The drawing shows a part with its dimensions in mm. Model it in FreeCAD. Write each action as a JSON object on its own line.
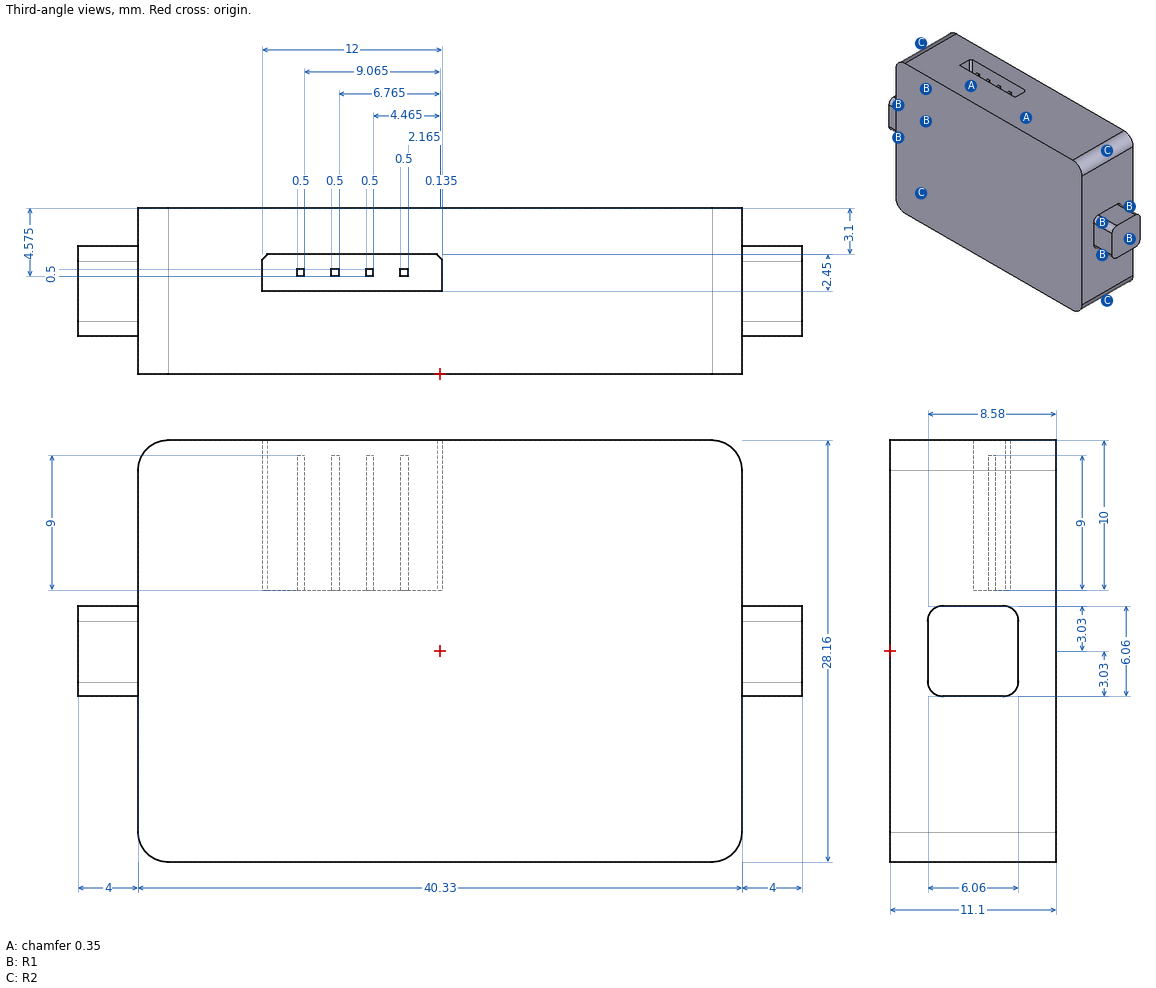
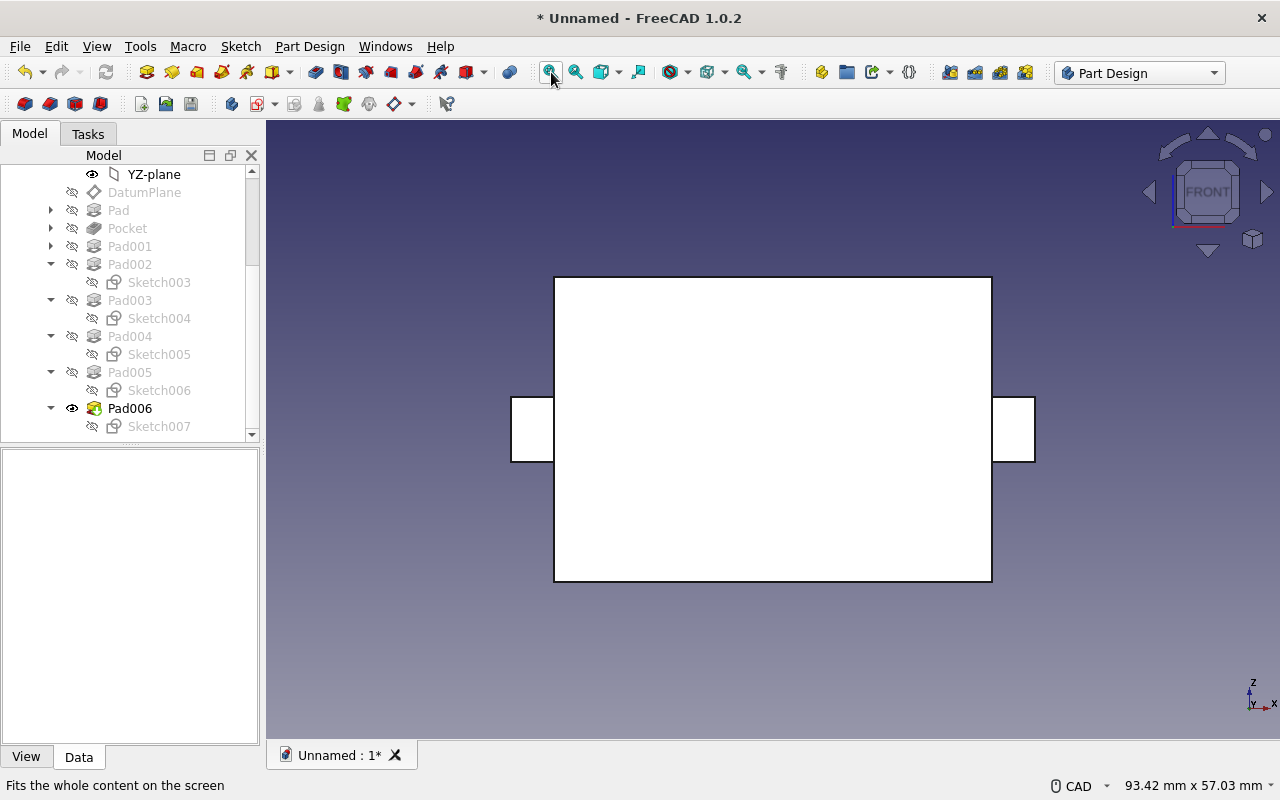
{"action": "key", "text": "3"}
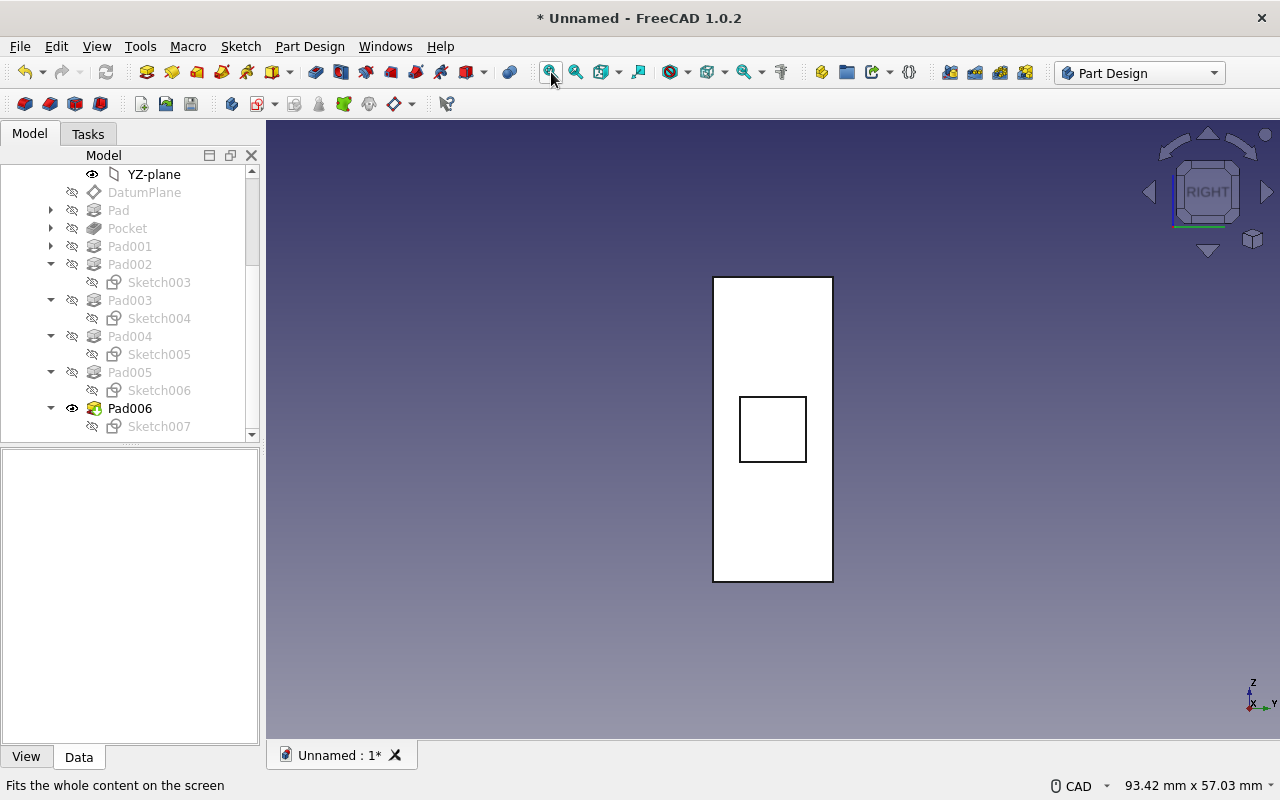
{"action": "key", "text": "5"}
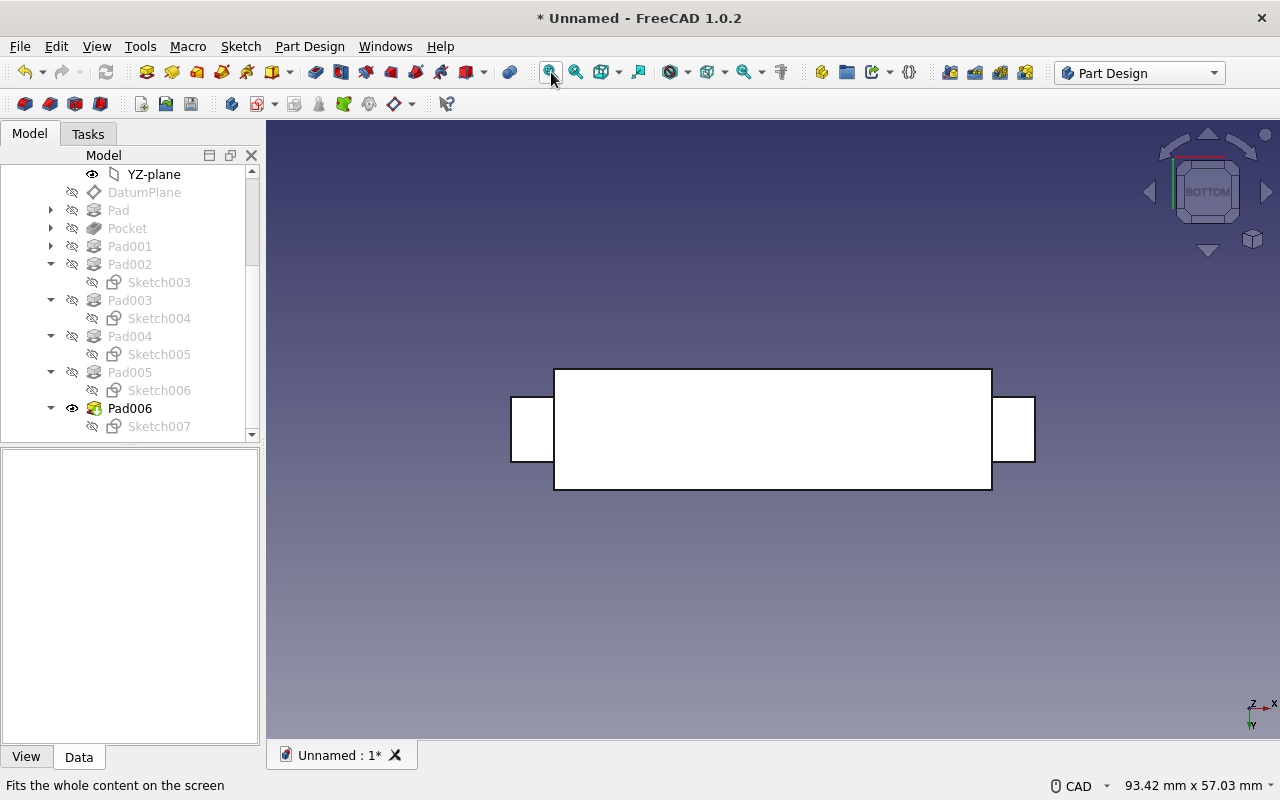
{"action": "key", "text": "4"}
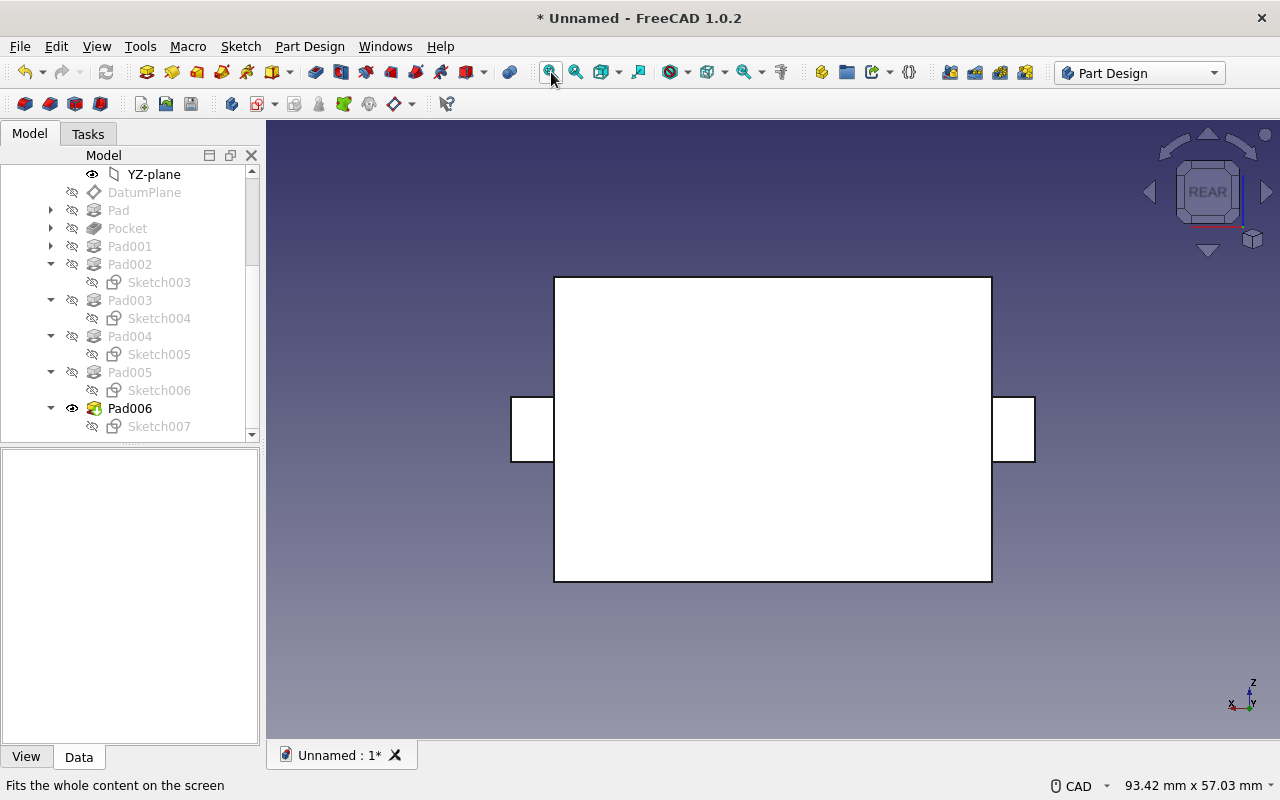
{"action": "key", "text": "6"}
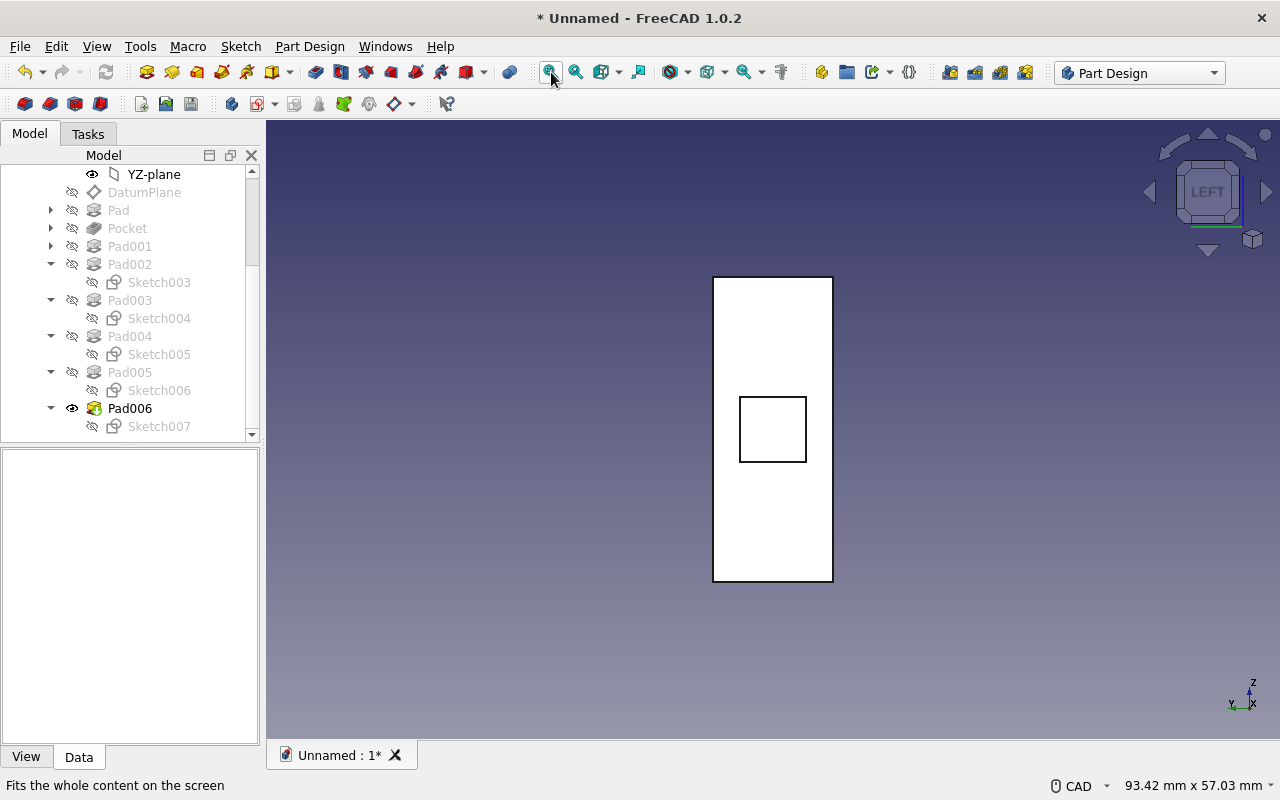
{"action": "key", "text": "v 3"}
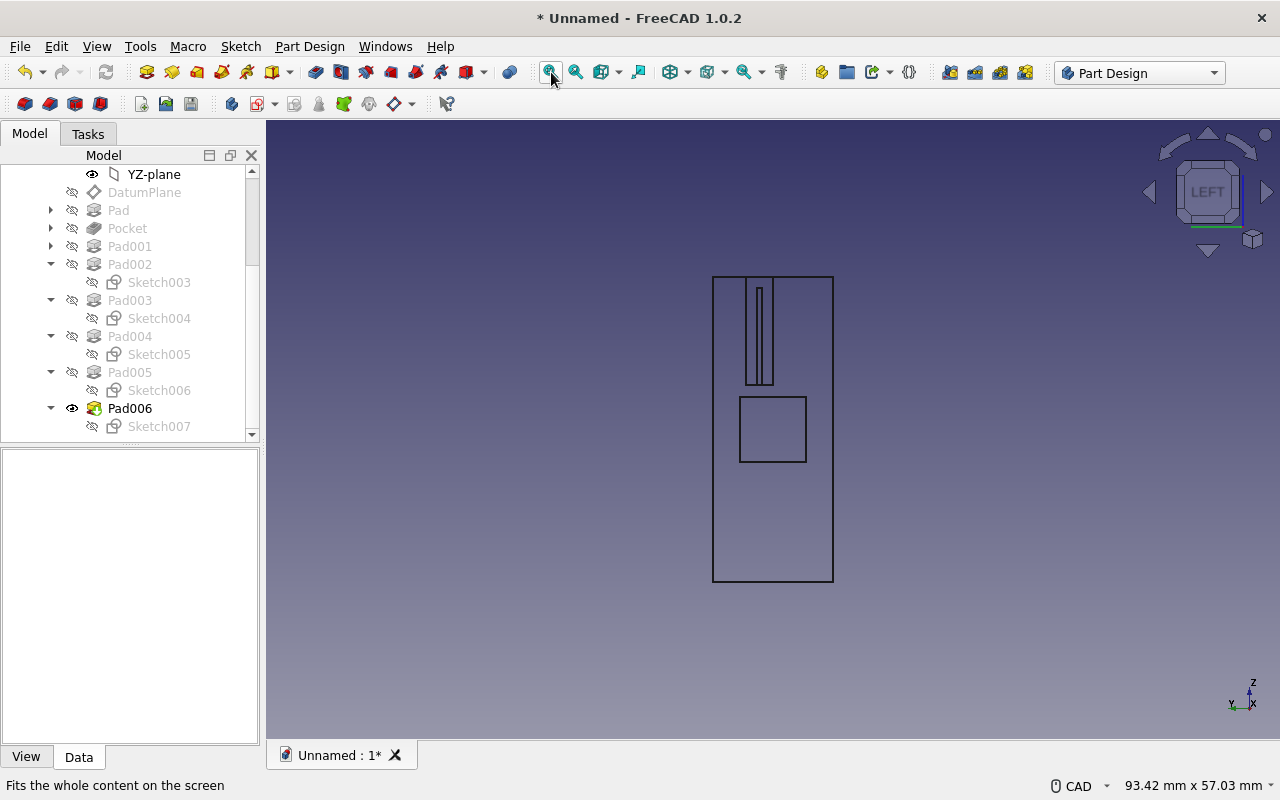
{"action": "key", "text": "0"}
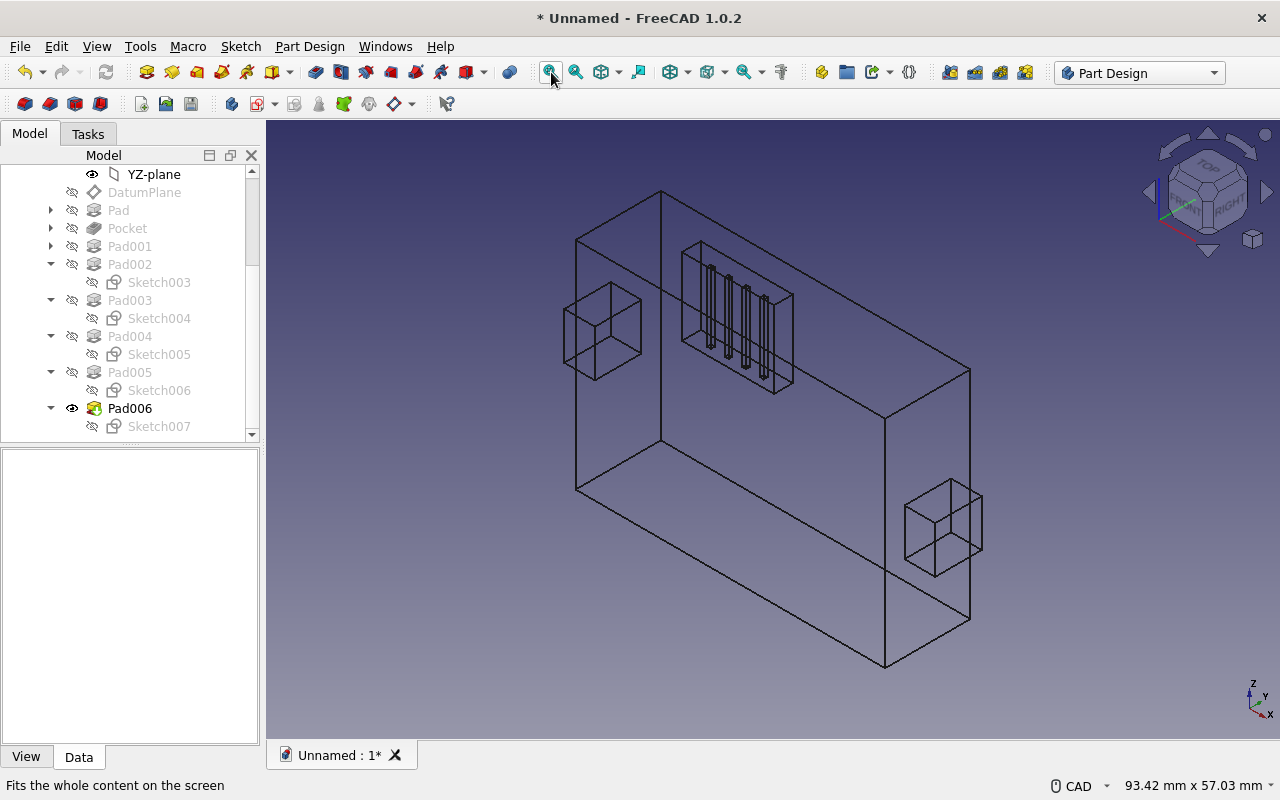
{"action": "left_click", "coordinate": [701, 285]}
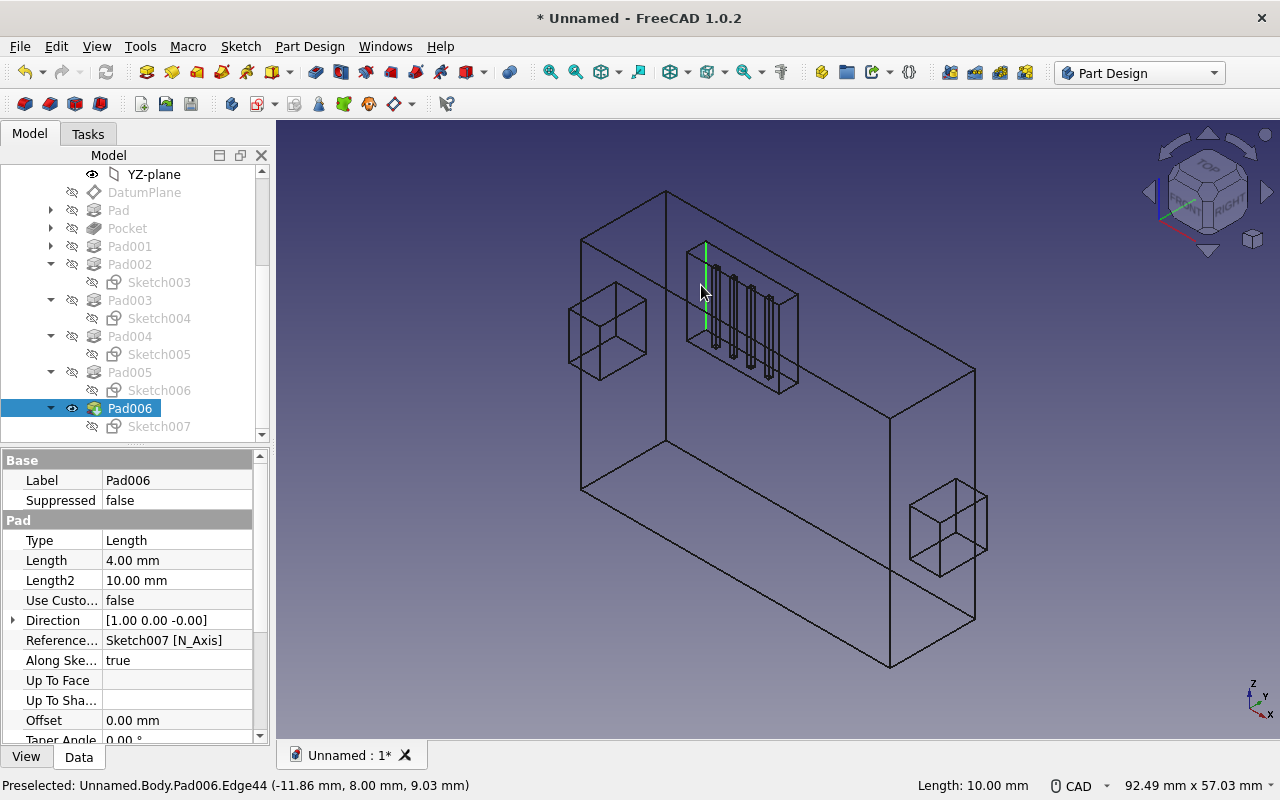
{"action": "left_click", "coordinate": [798, 338], "text": "ctrl"}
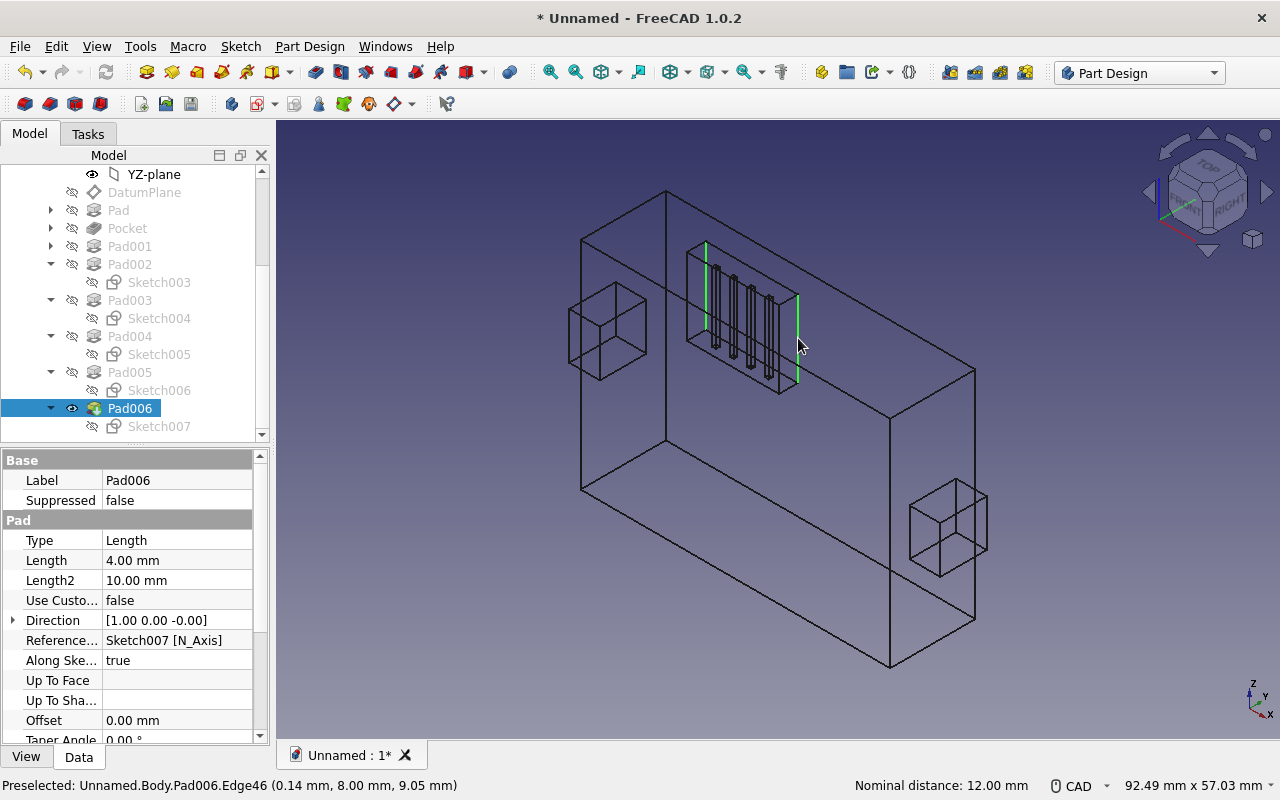
{"action": "key", "text": "v 1"}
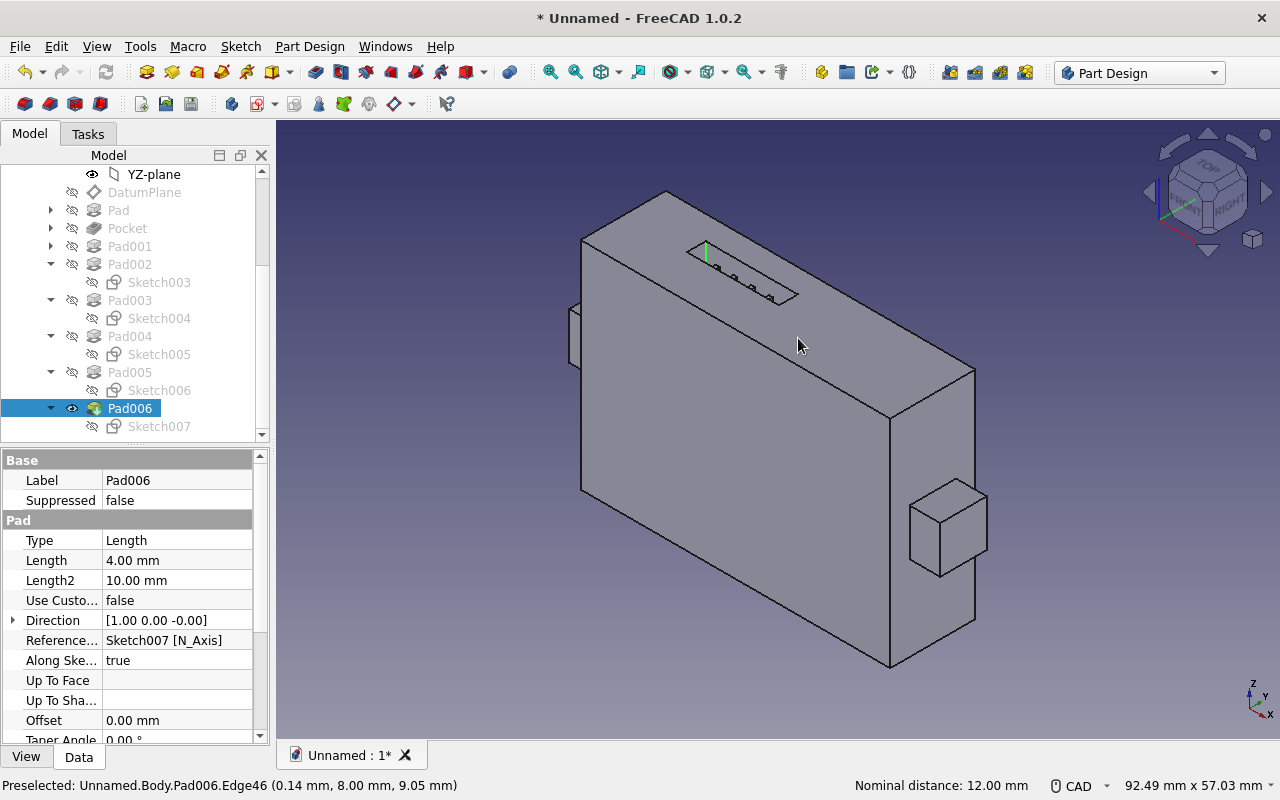
{"action": "left_click", "coordinate": [50, 104]}